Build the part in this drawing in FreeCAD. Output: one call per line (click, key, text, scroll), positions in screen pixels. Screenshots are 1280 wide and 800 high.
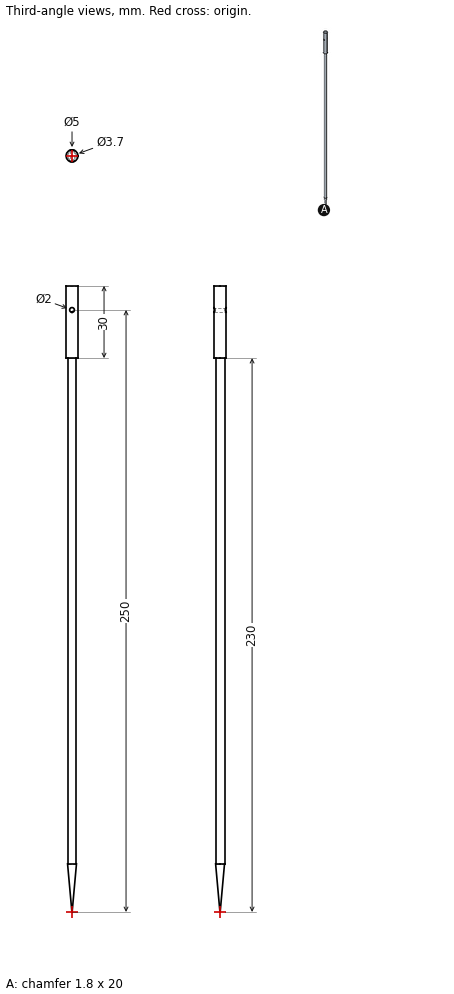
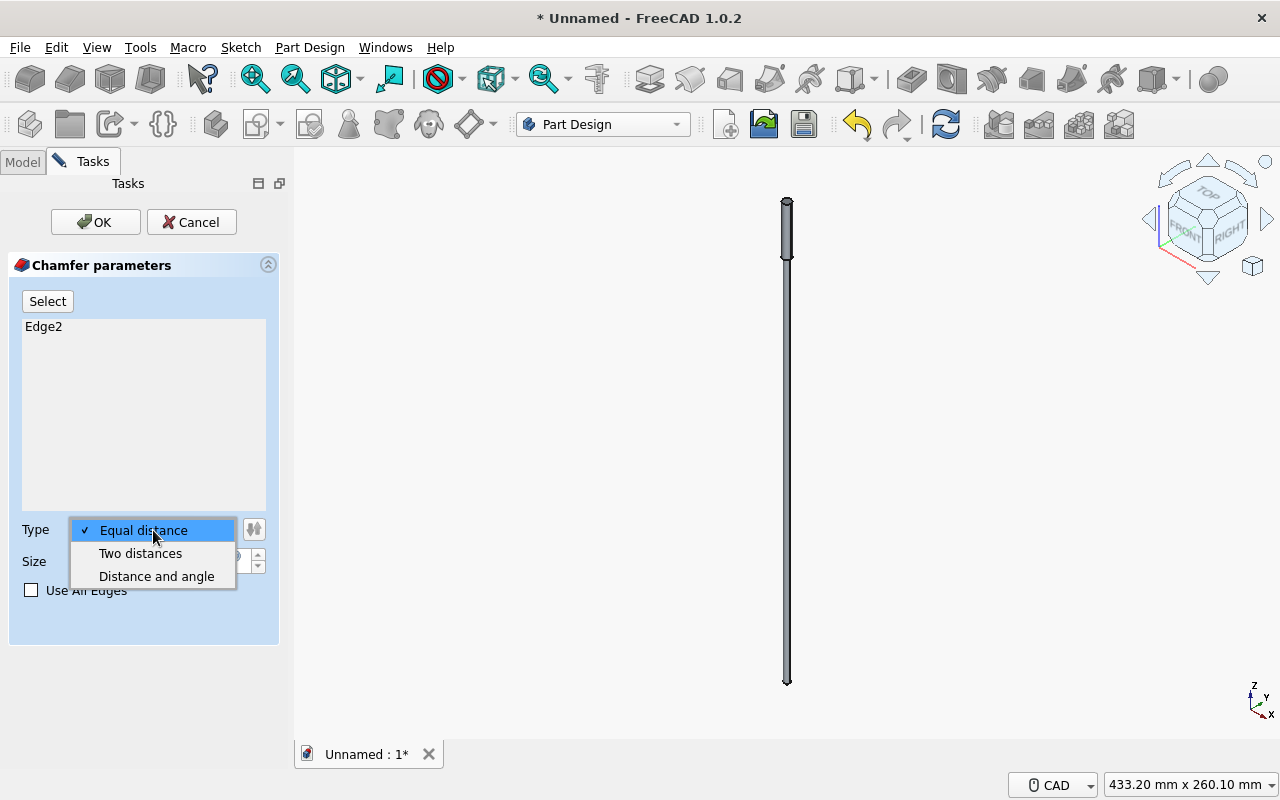
click(152, 554)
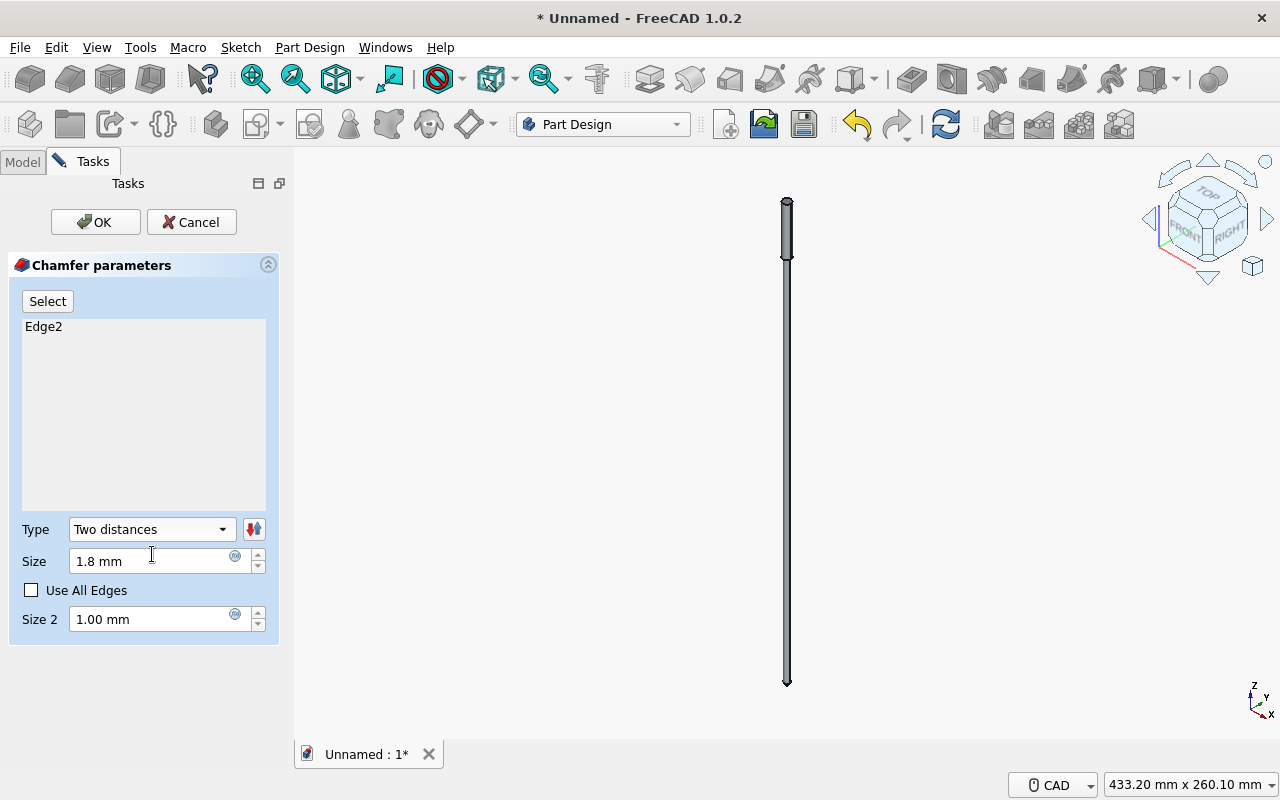
triple_click(160, 619)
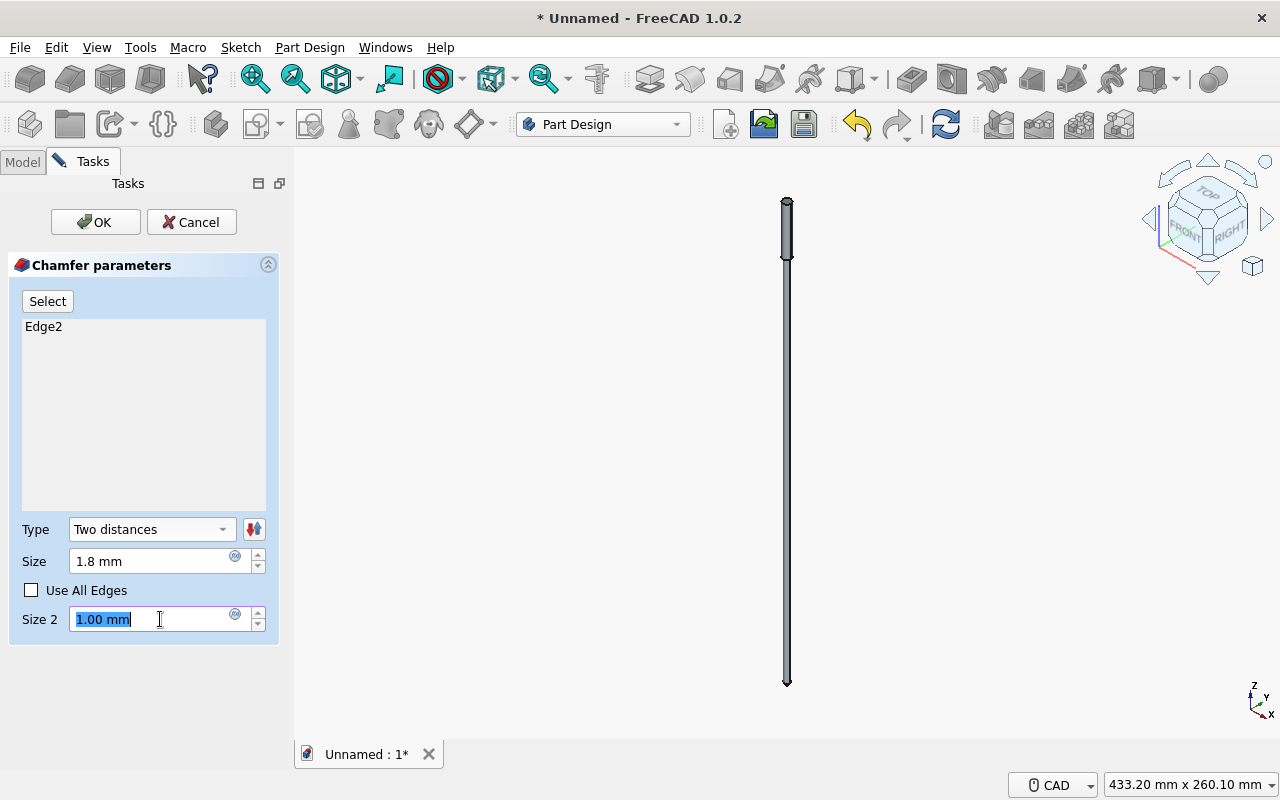
text(20)
key(Tab)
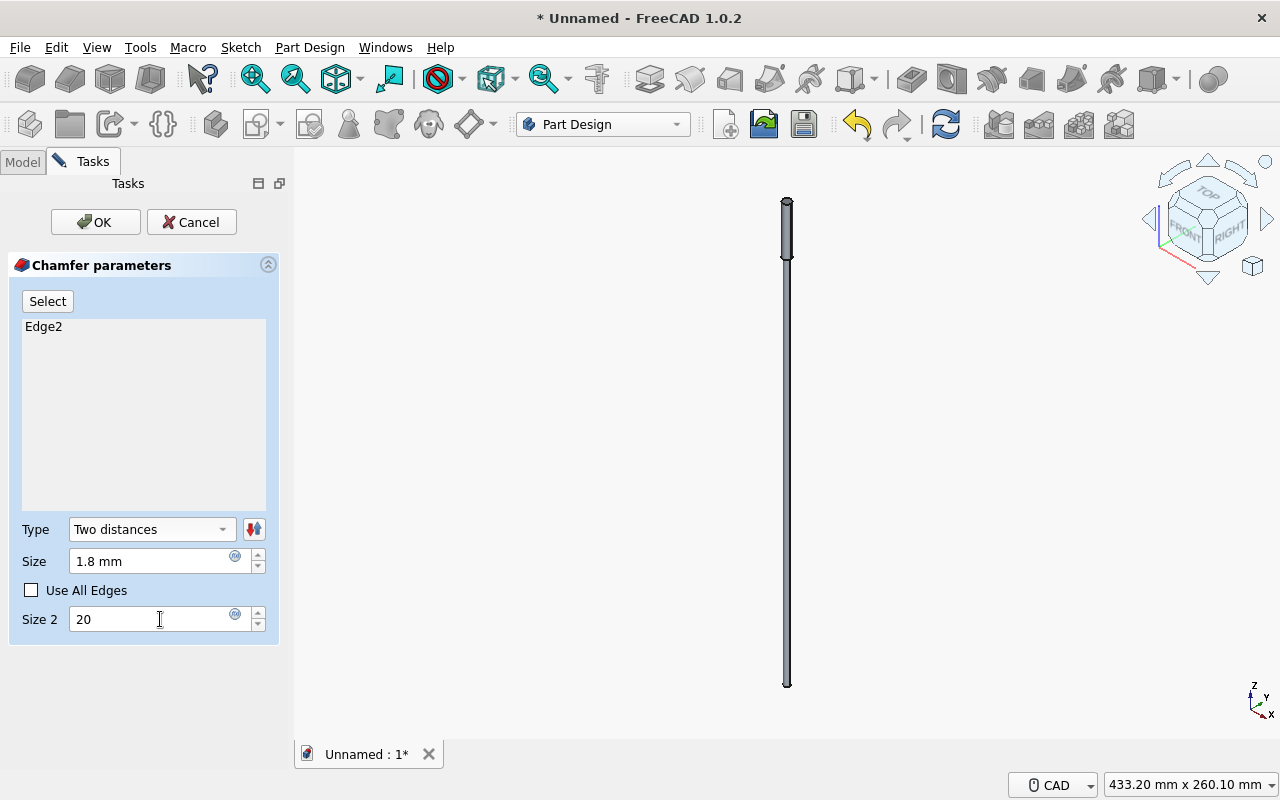
click(254, 530)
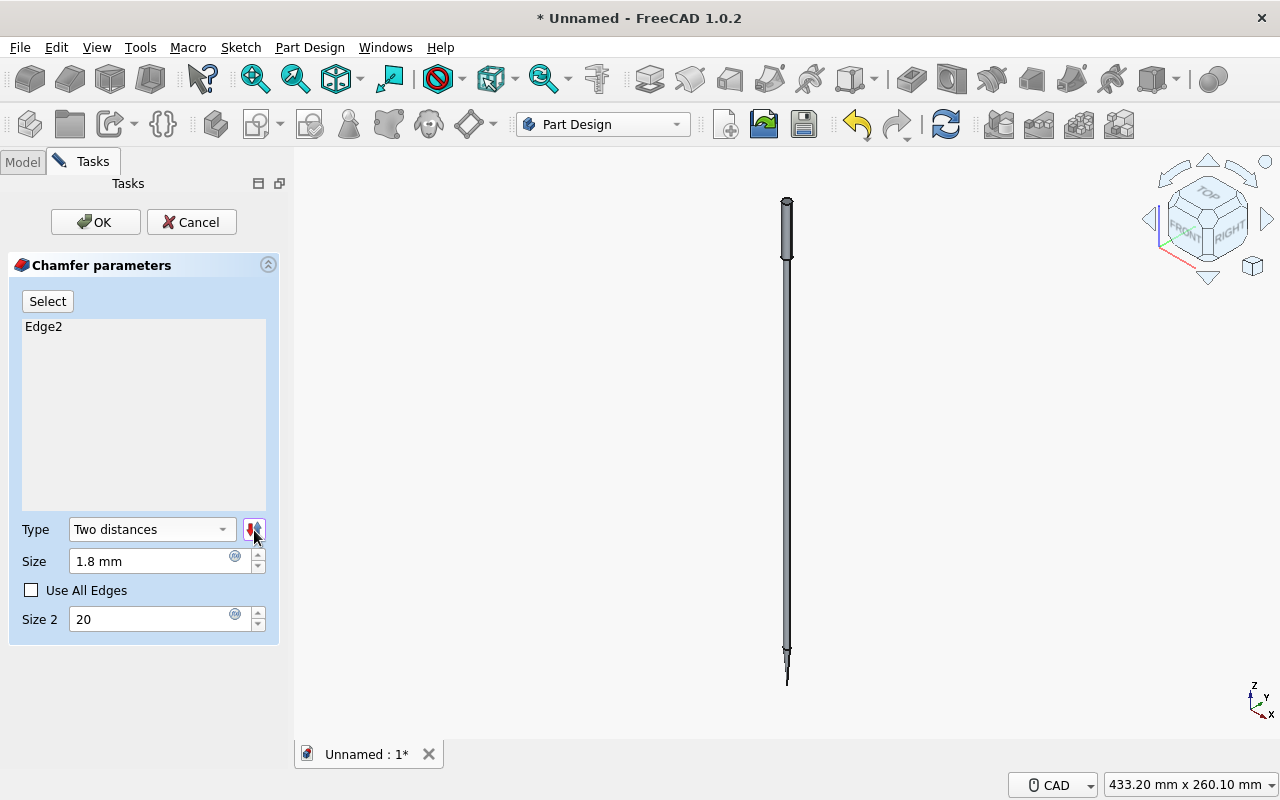
click(96, 222)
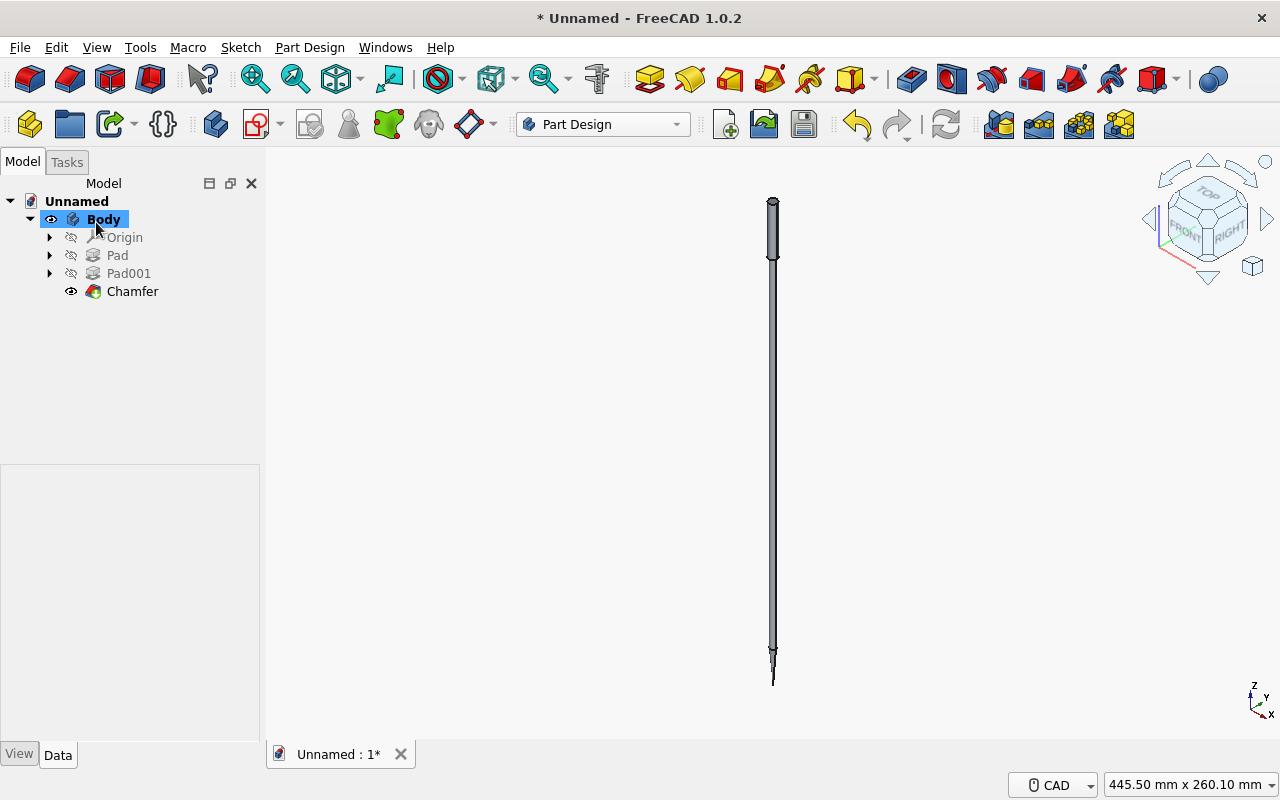
click(256, 124)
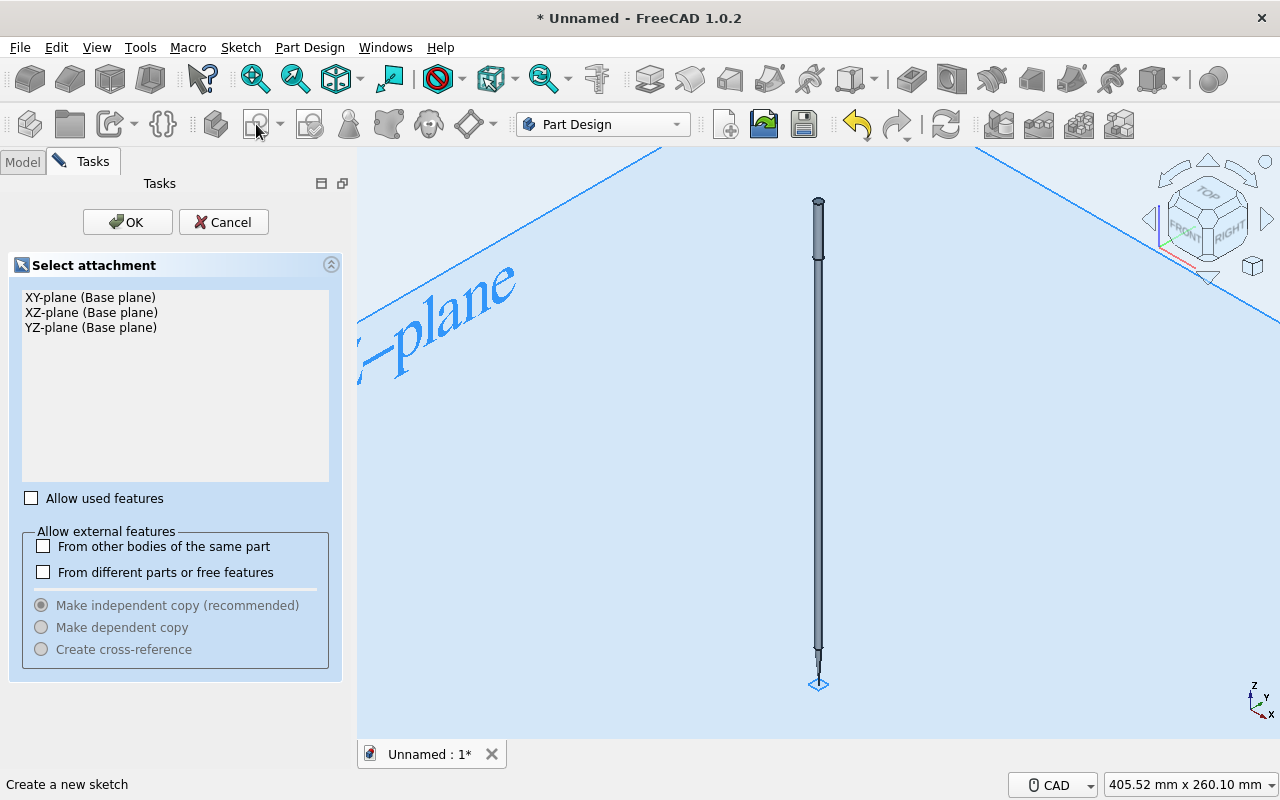
click(82, 312)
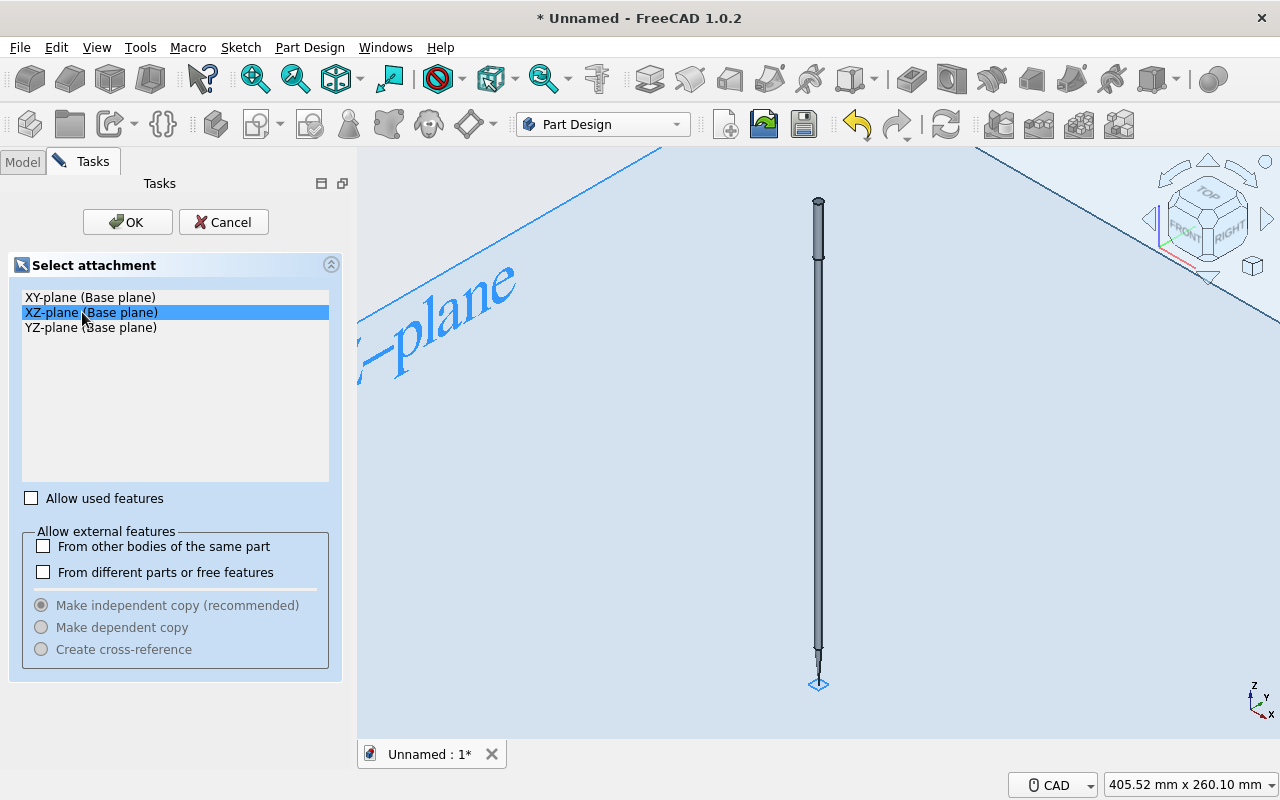
click(128, 222)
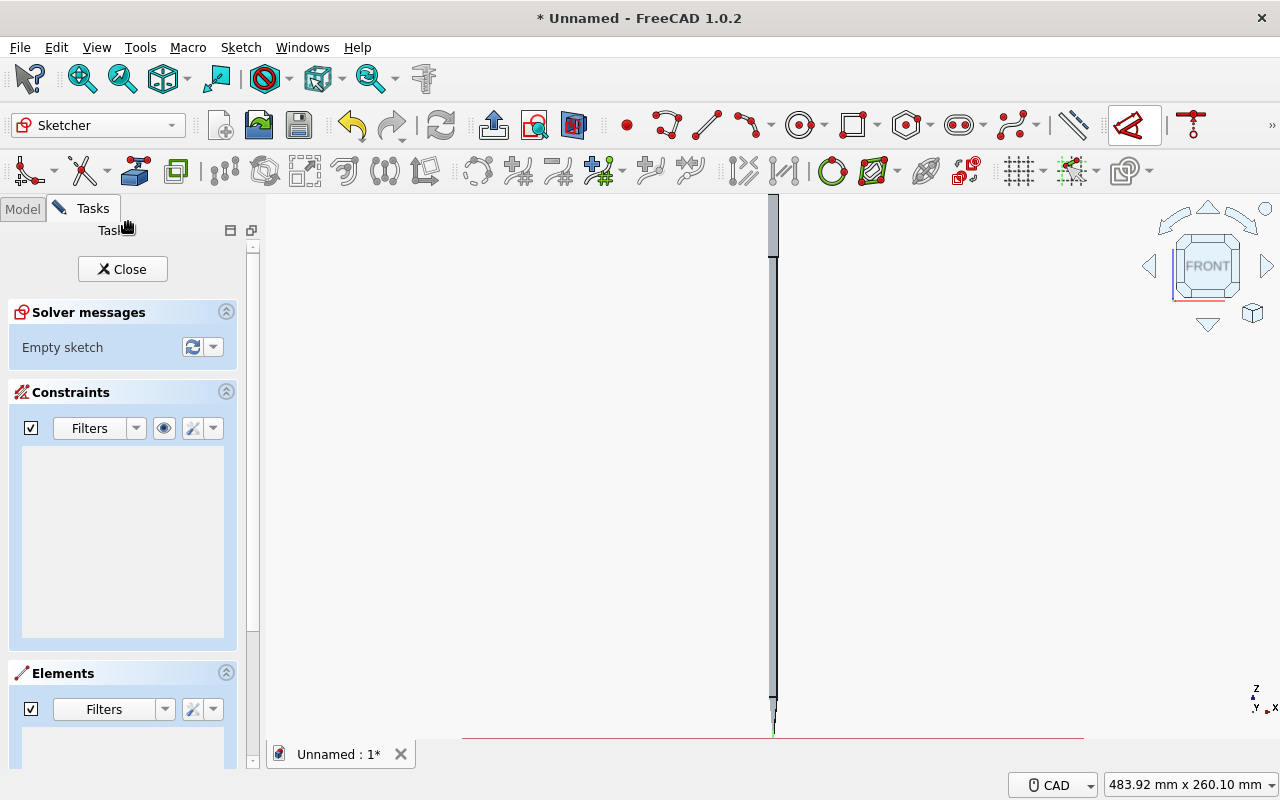
key(q)
key(s)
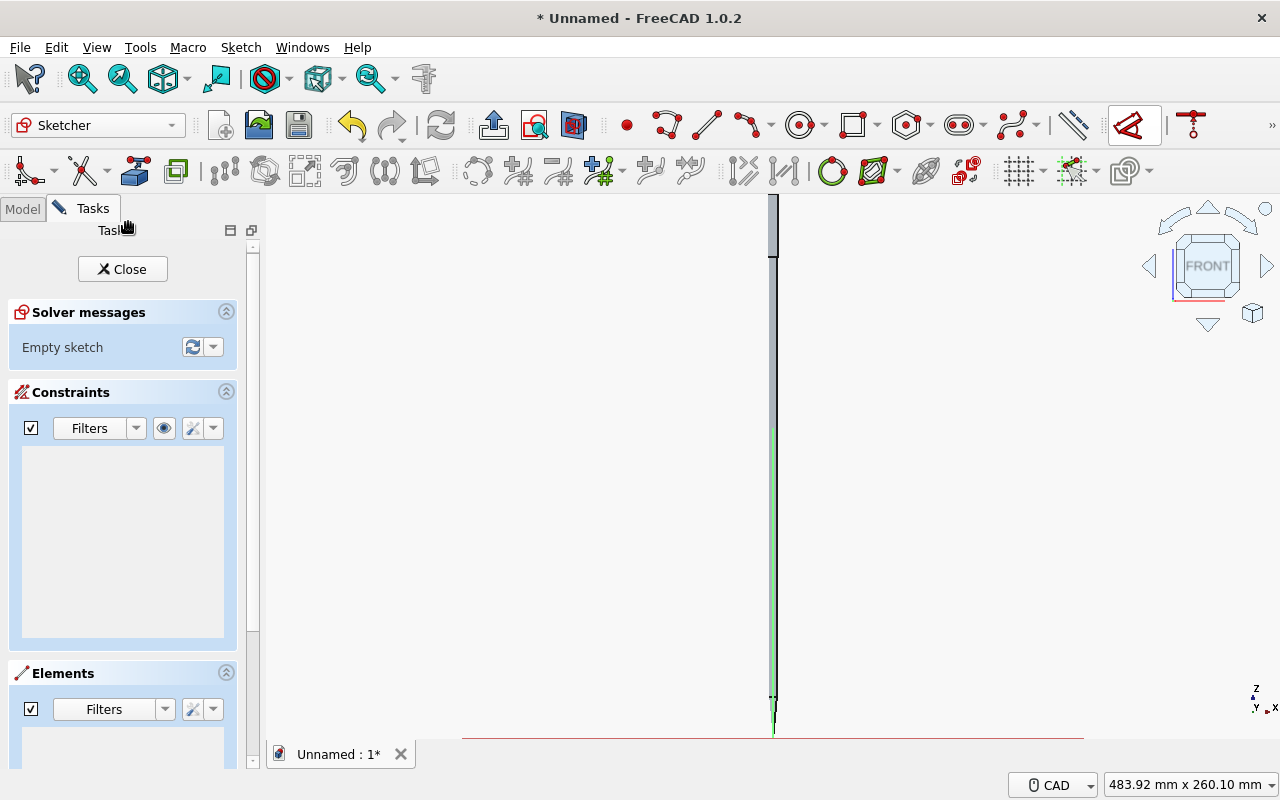
scroll(704, 466, down, 5)